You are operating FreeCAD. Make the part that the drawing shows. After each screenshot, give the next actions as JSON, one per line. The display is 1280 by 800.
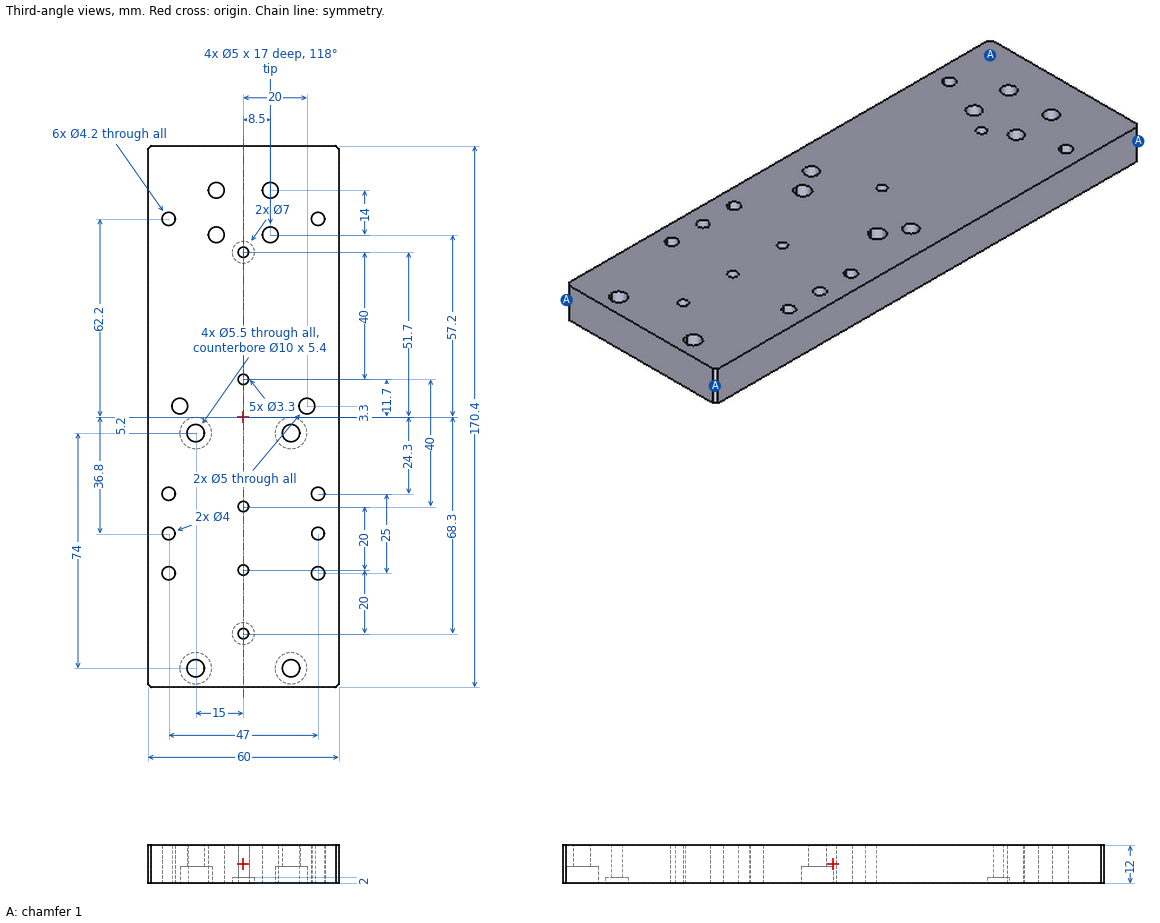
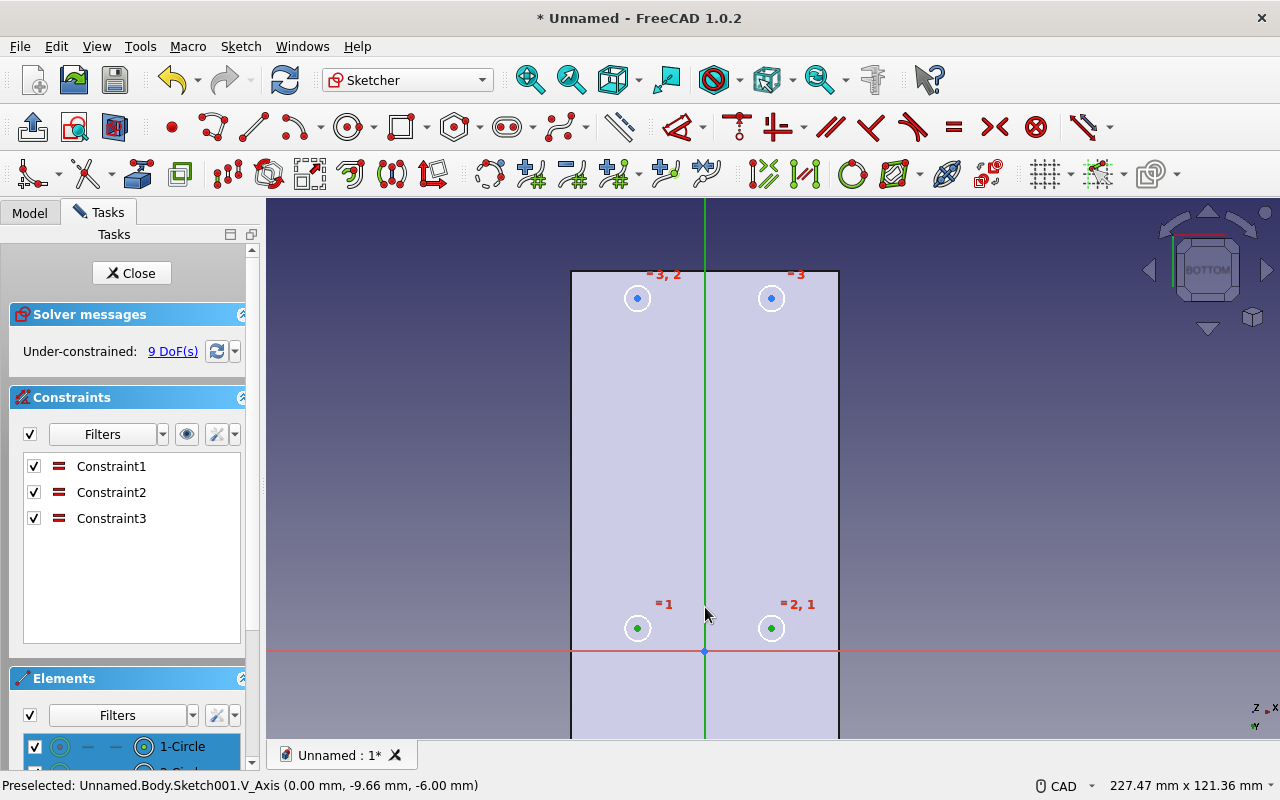
{"action": "left_click", "coordinate": [995, 128]}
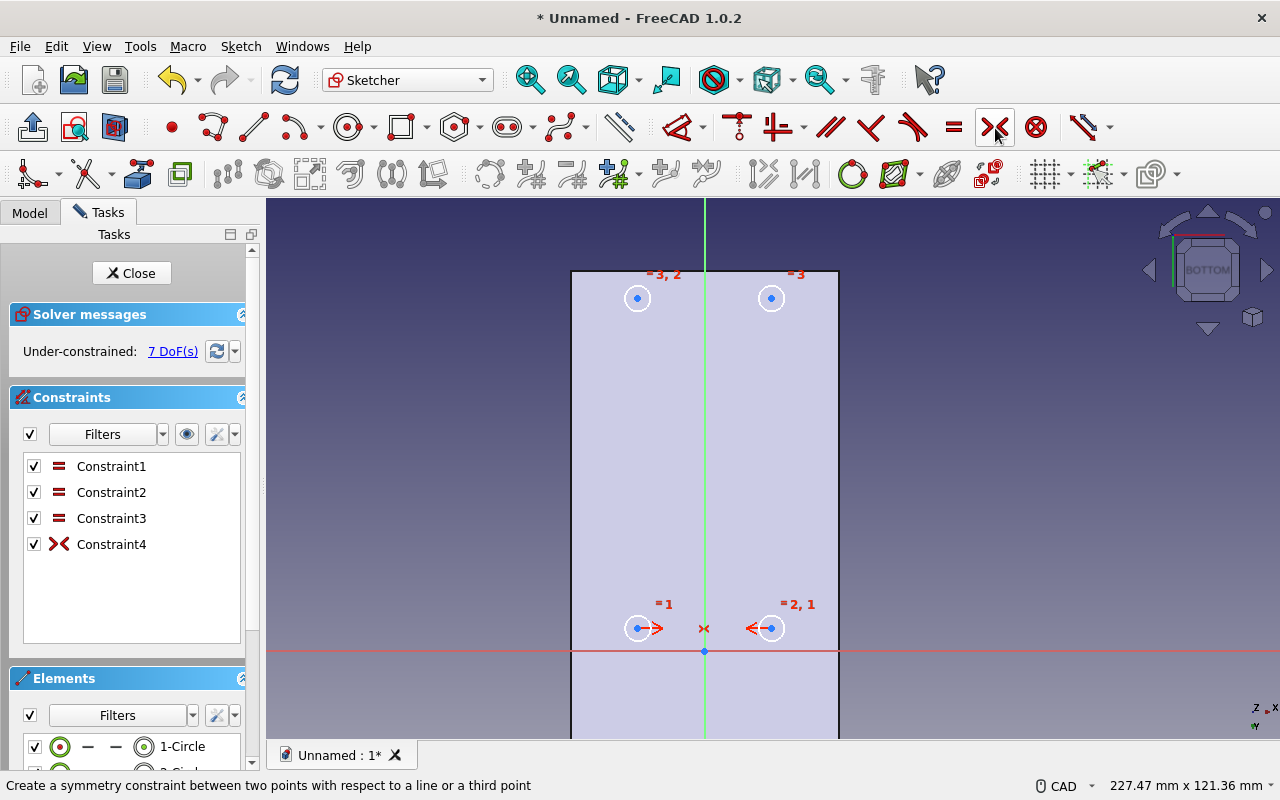
{"action": "left_click", "coordinate": [638, 299]}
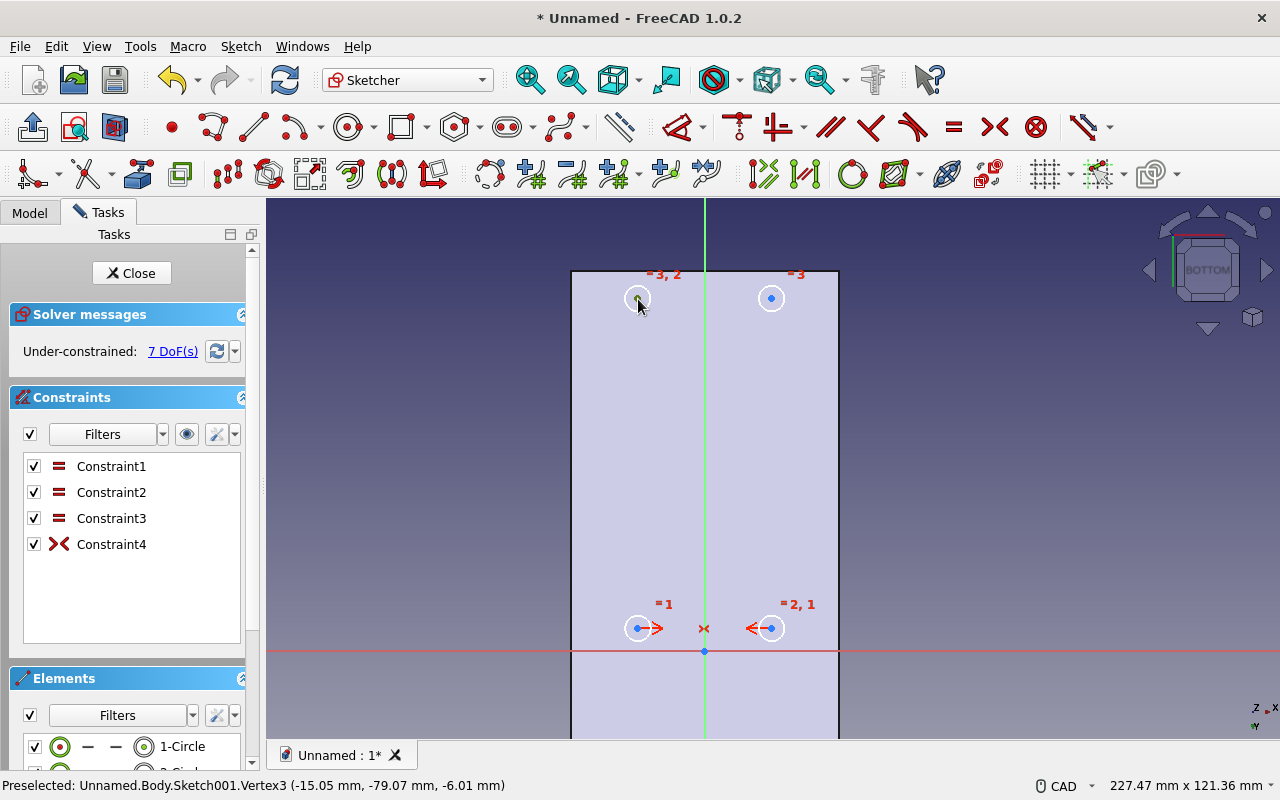
{"action": "left_click", "coordinate": [772, 299]}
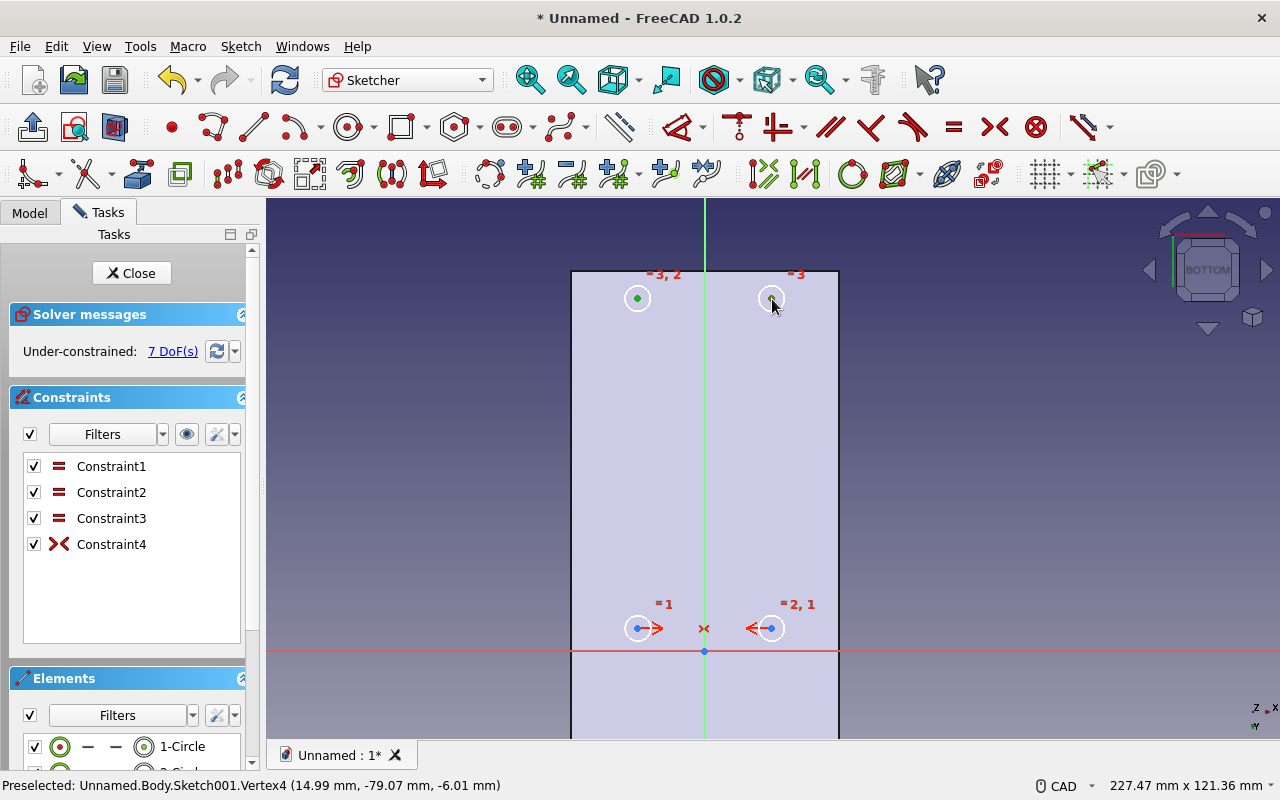
{"action": "left_click", "coordinate": [705, 607]}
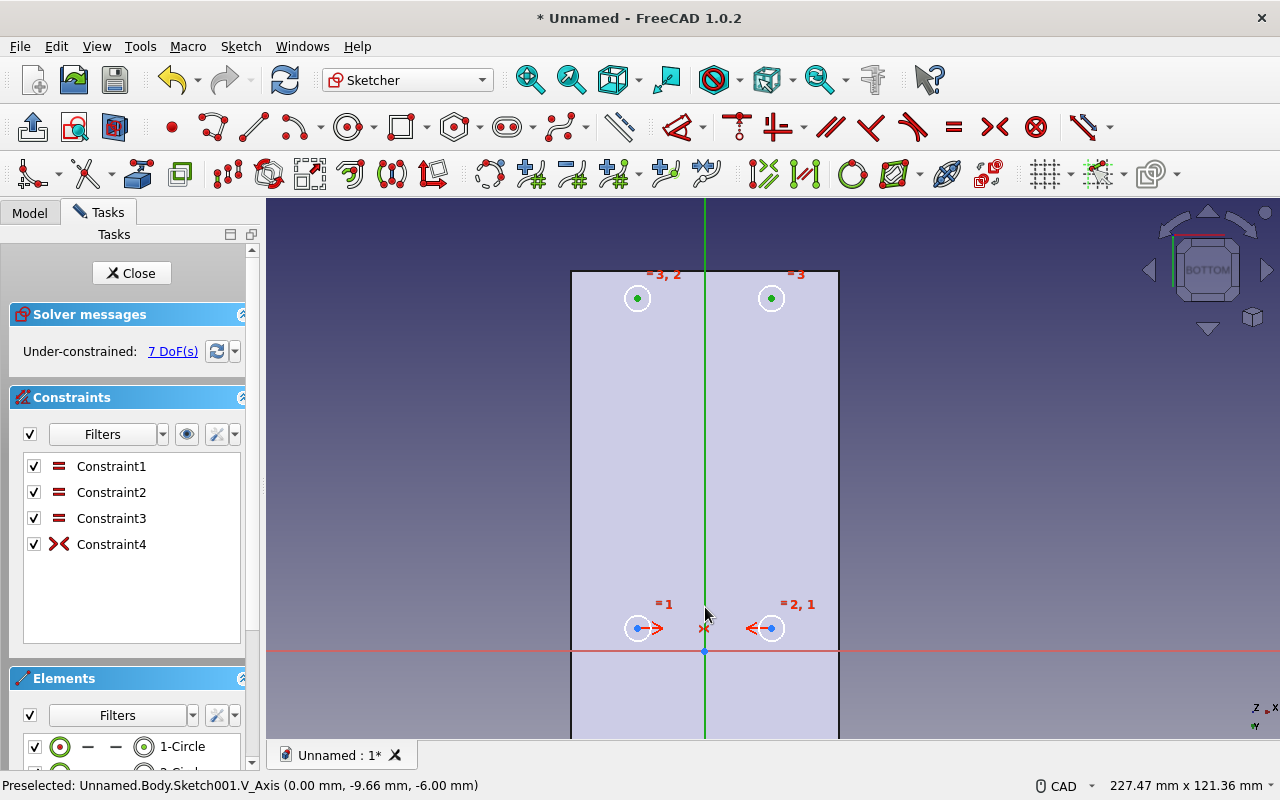
{"action": "left_click", "coordinate": [995, 128]}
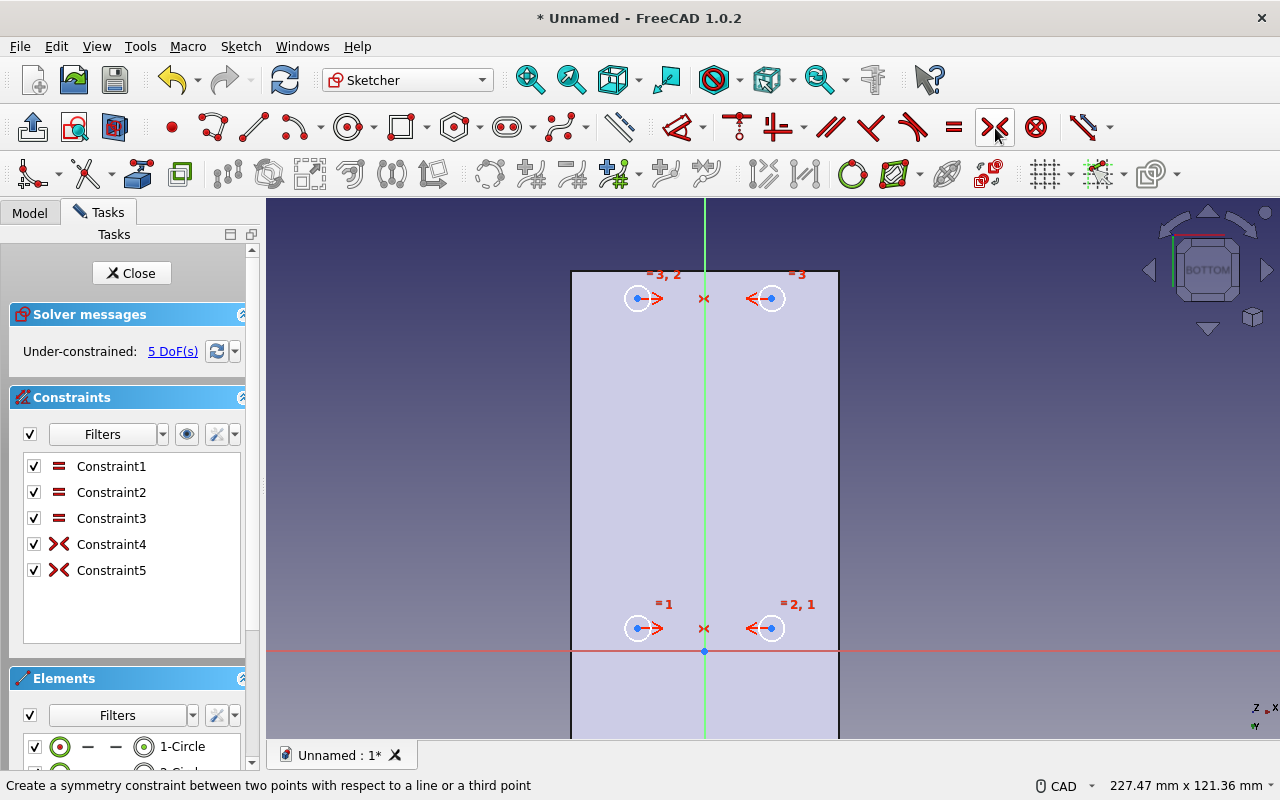
{"action": "left_click", "coordinate": [676, 128]}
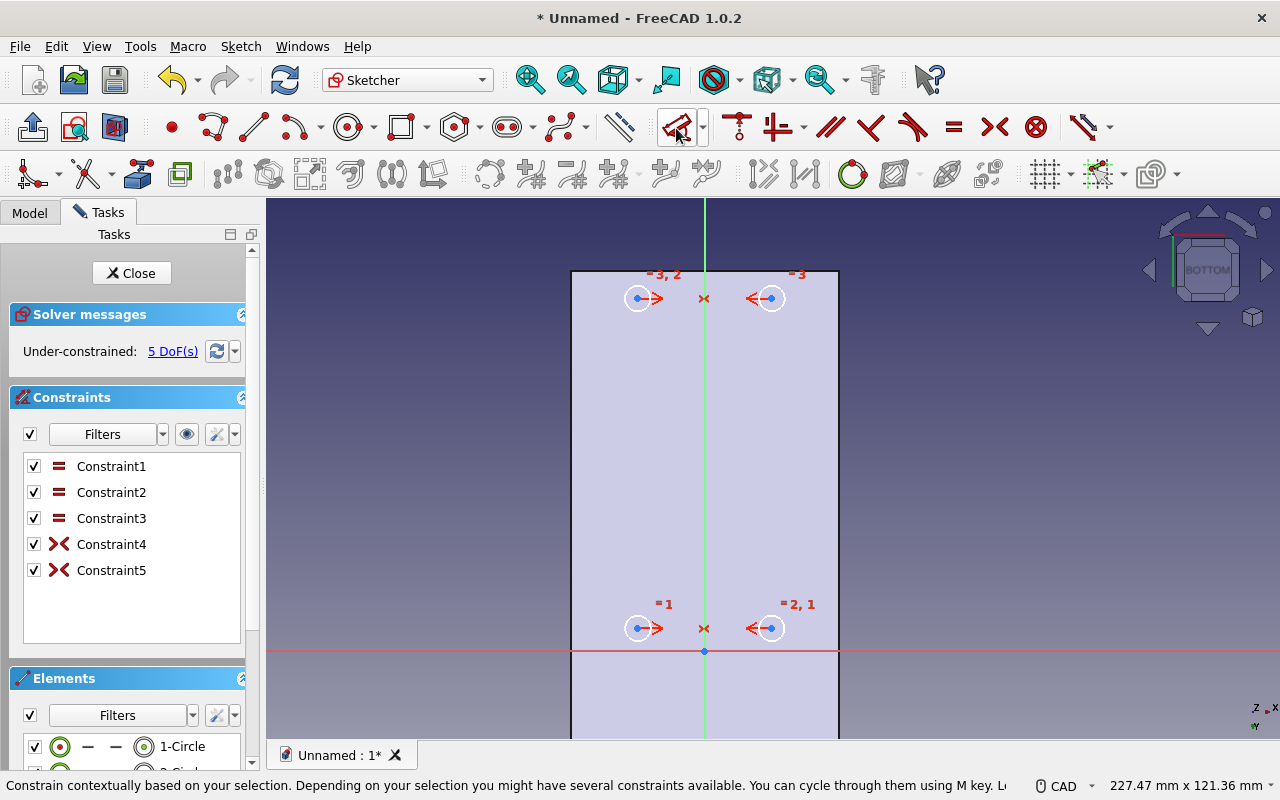
{"action": "scroll", "coordinate": [647, 619], "scroll_direction": "up", "scroll_amount": 3}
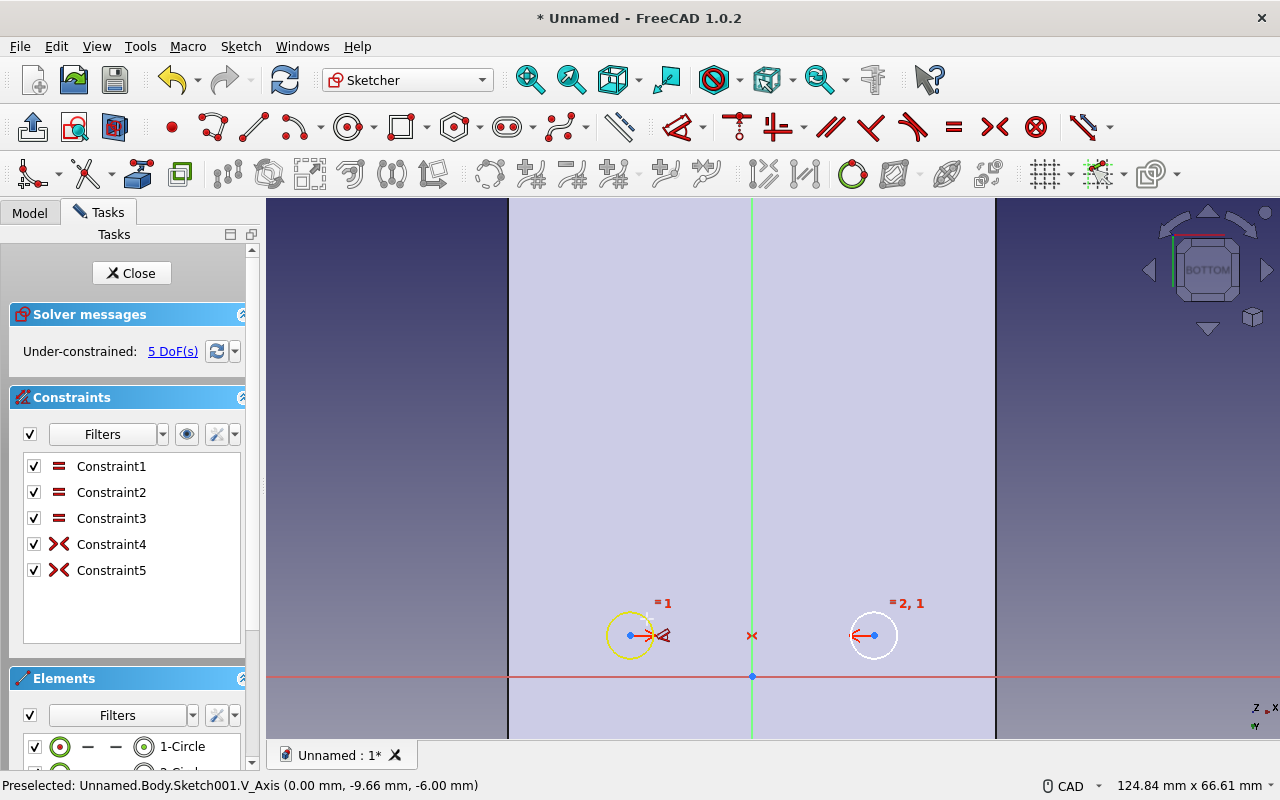
{"action": "left_click", "coordinate": [646, 619]}
{"action": "left_click", "coordinate": [668, 596]}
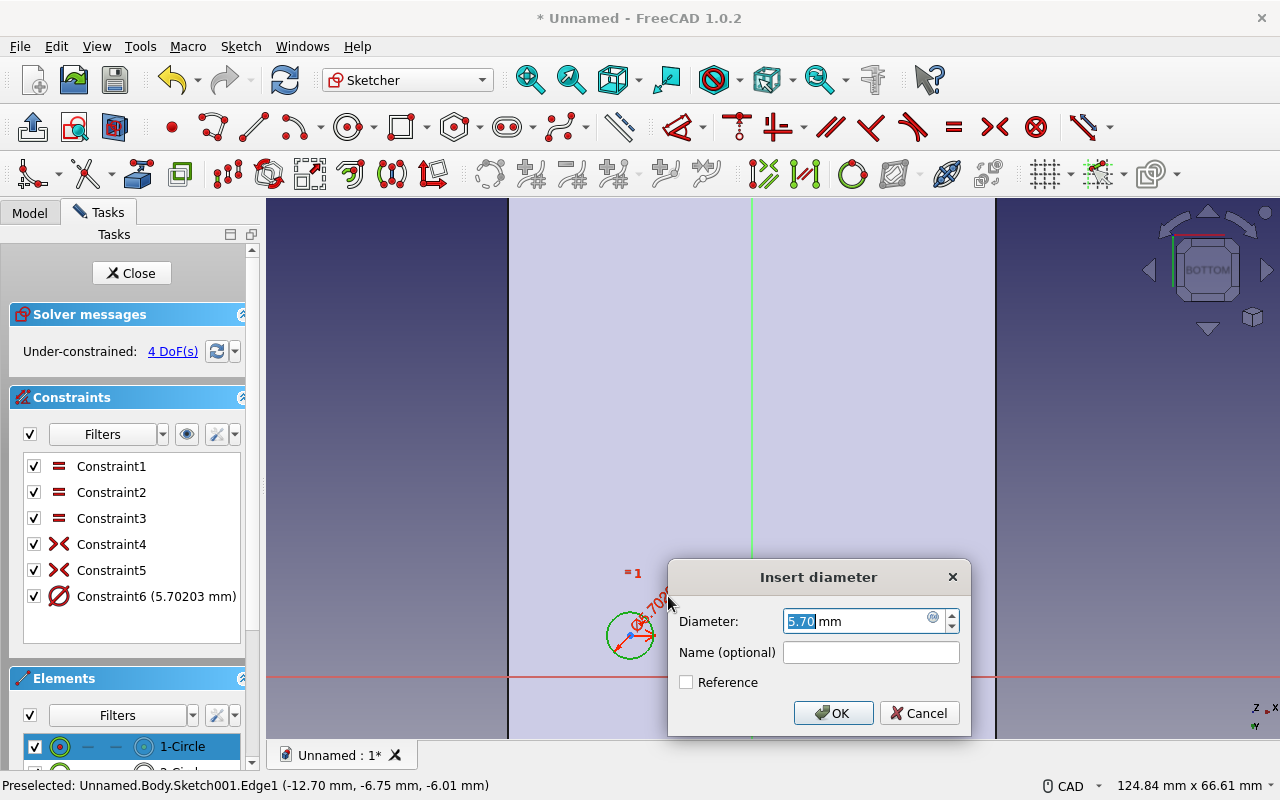
{"action": "type", "text": "5.5"}
{"action": "key", "text": "Return"}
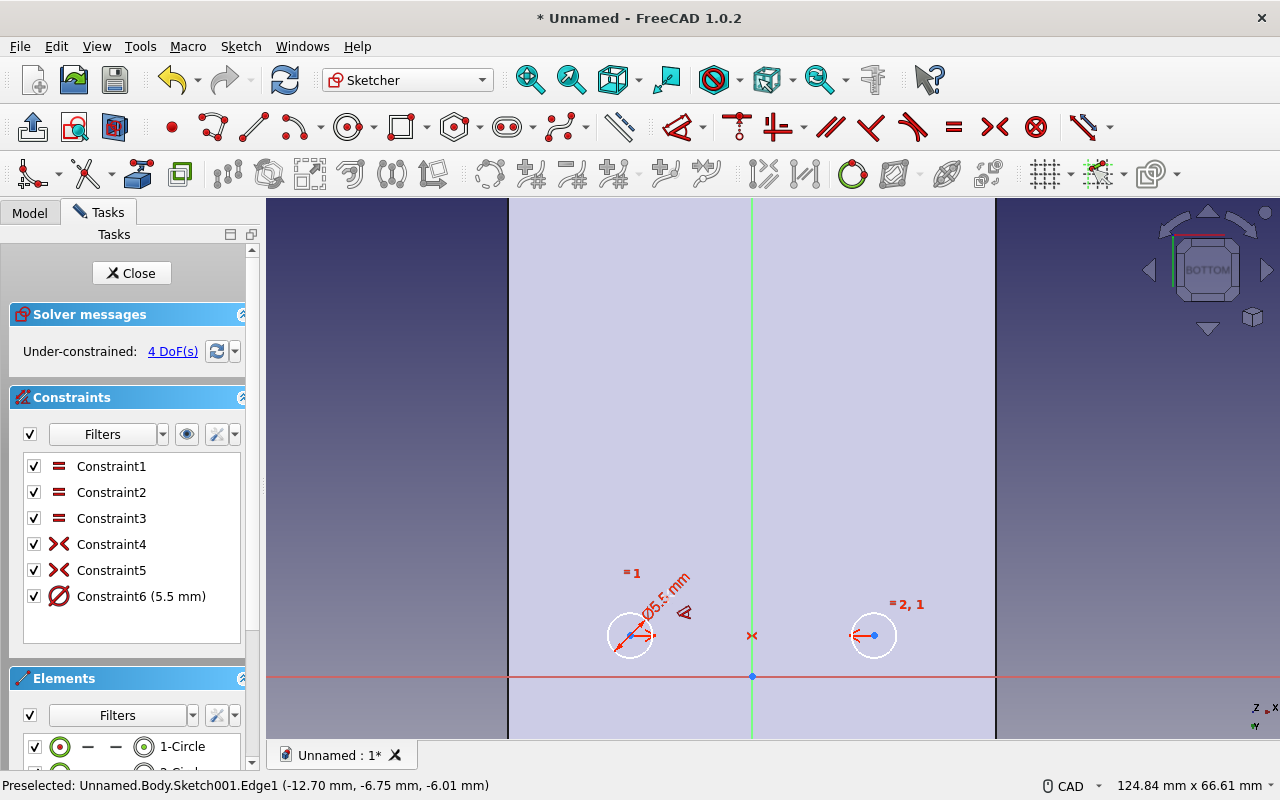
{"action": "left_click", "coordinate": [630, 636]}
{"action": "left_click", "coordinate": [691, 711]}